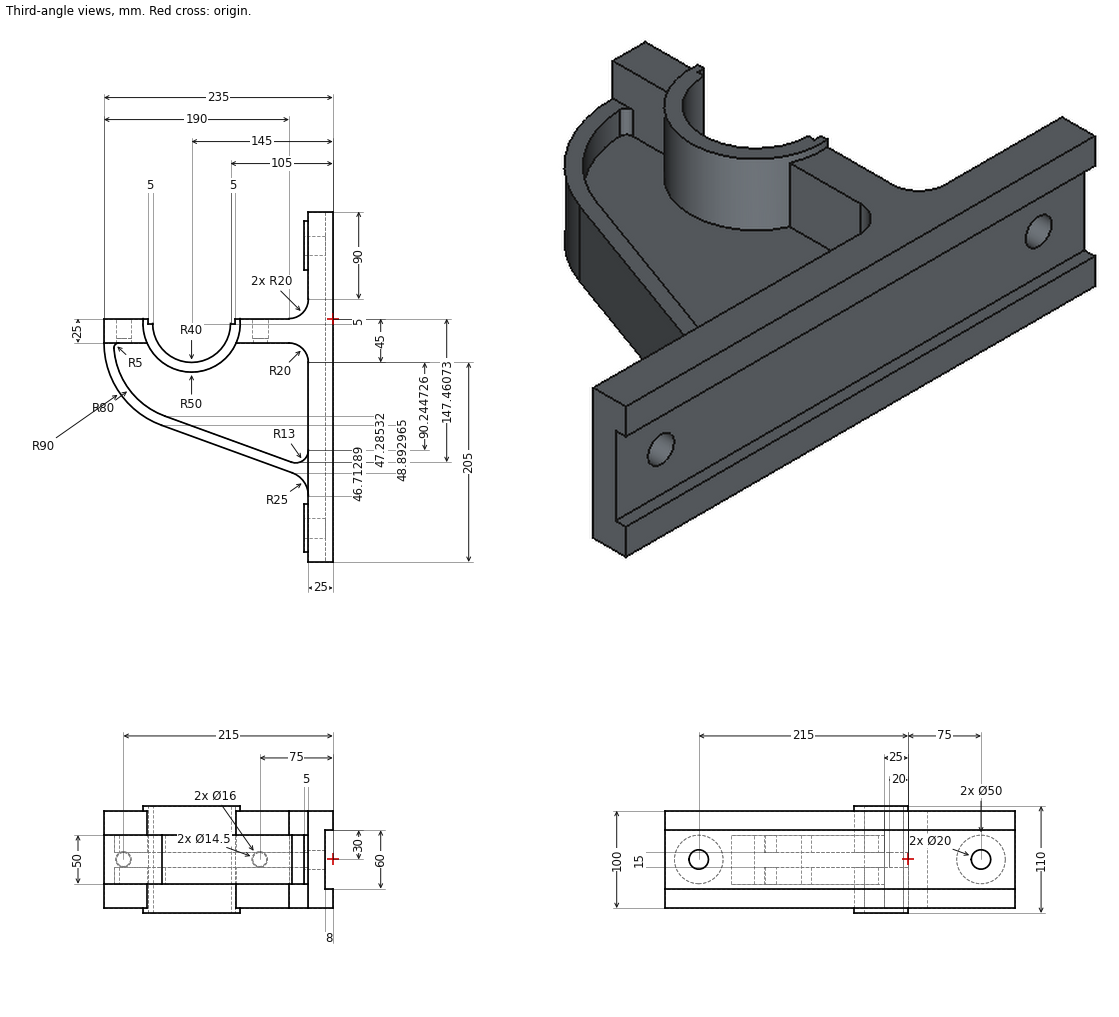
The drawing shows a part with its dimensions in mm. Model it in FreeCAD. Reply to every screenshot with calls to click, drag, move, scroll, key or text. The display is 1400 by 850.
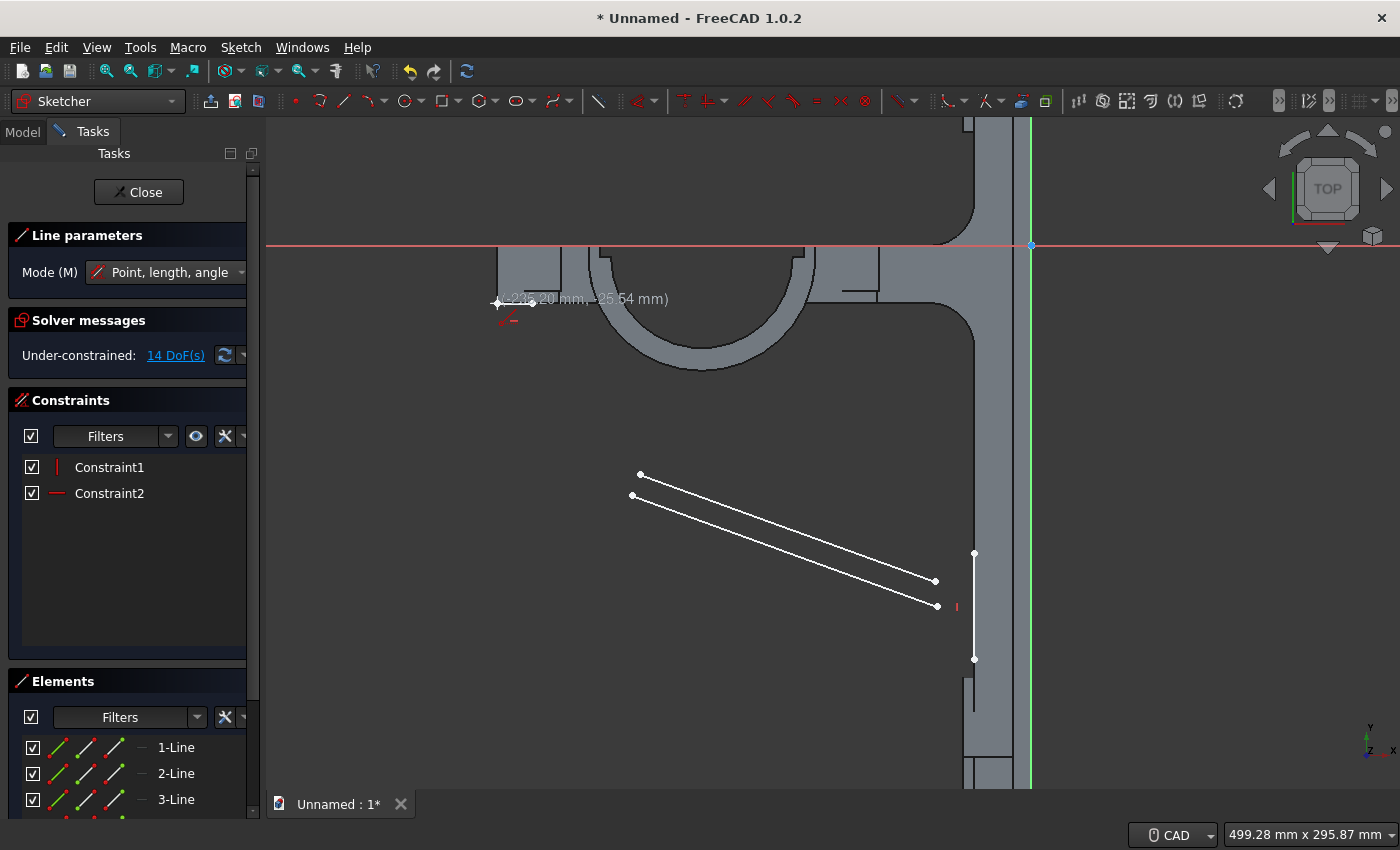
click(368, 102)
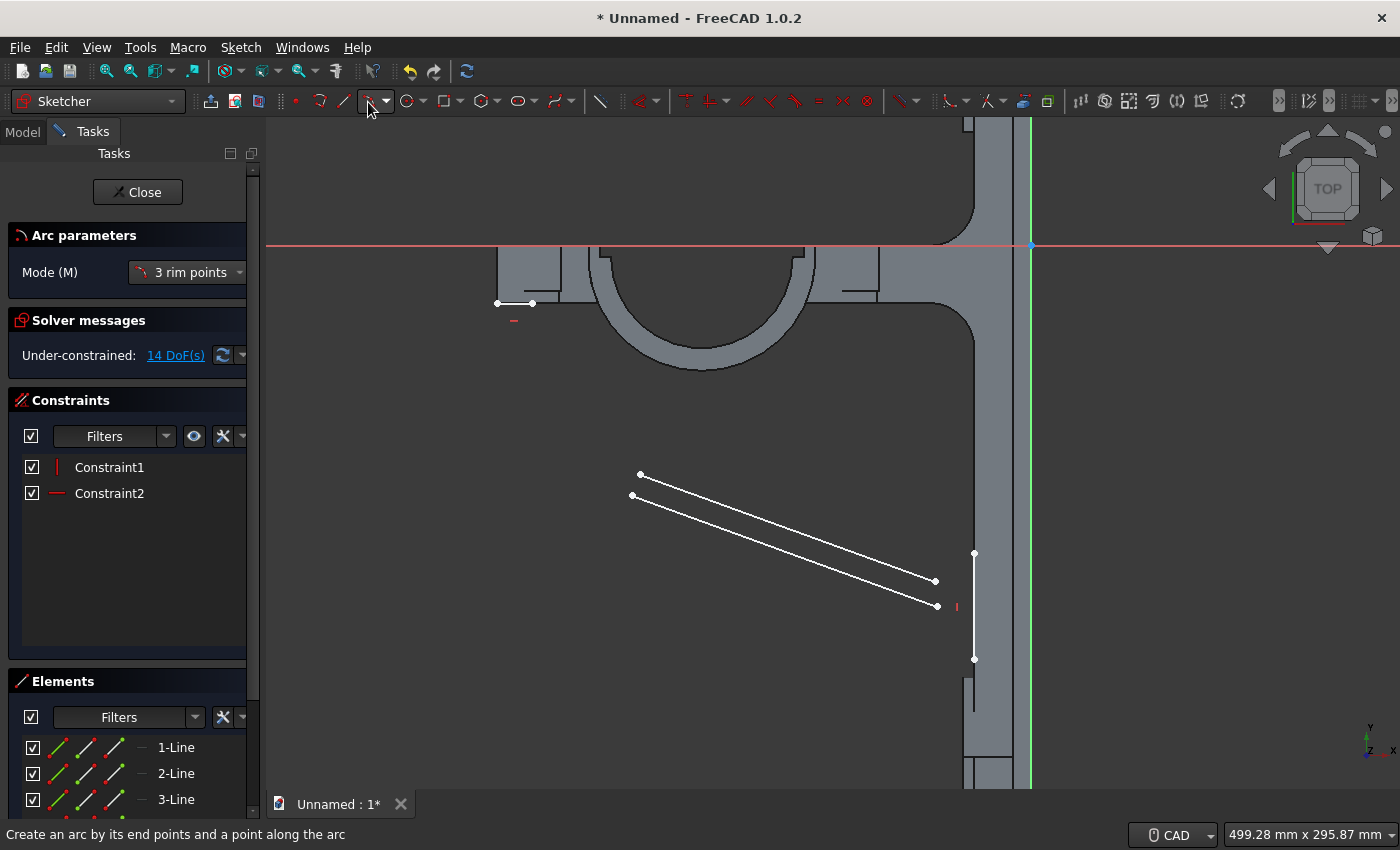
click(937, 607)
click(974, 660)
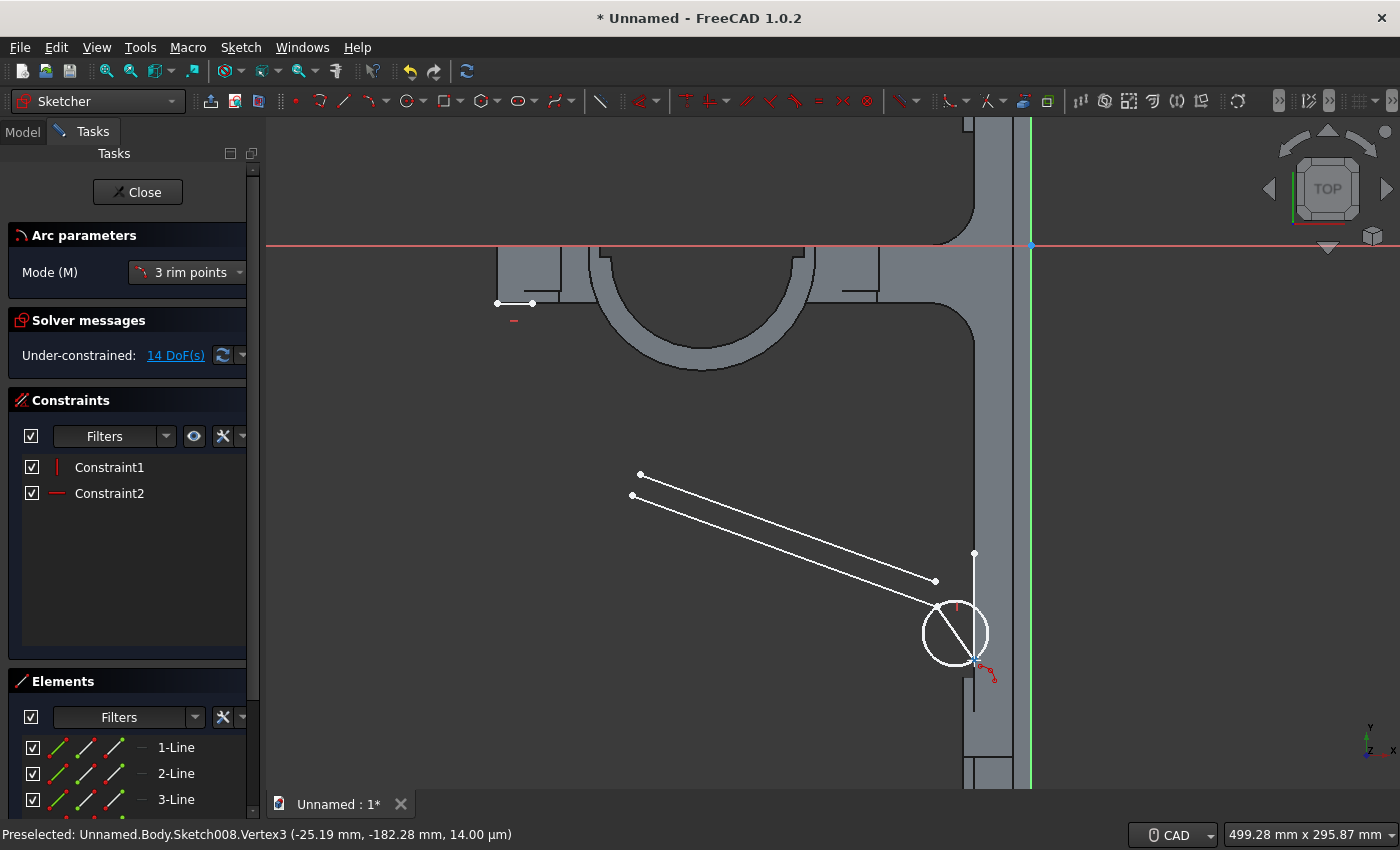
scroll(964, 627, up, 3)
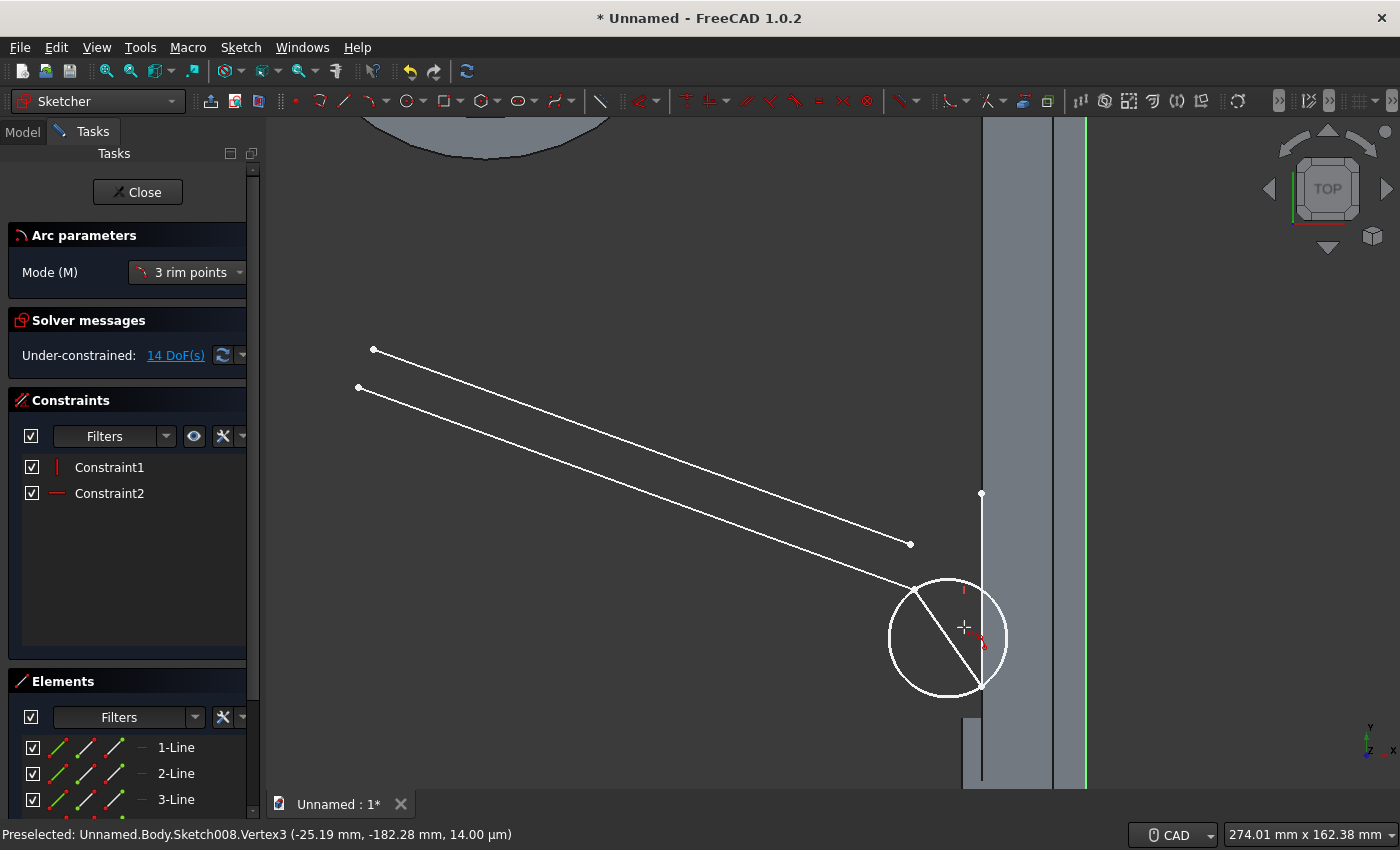
click(964, 626)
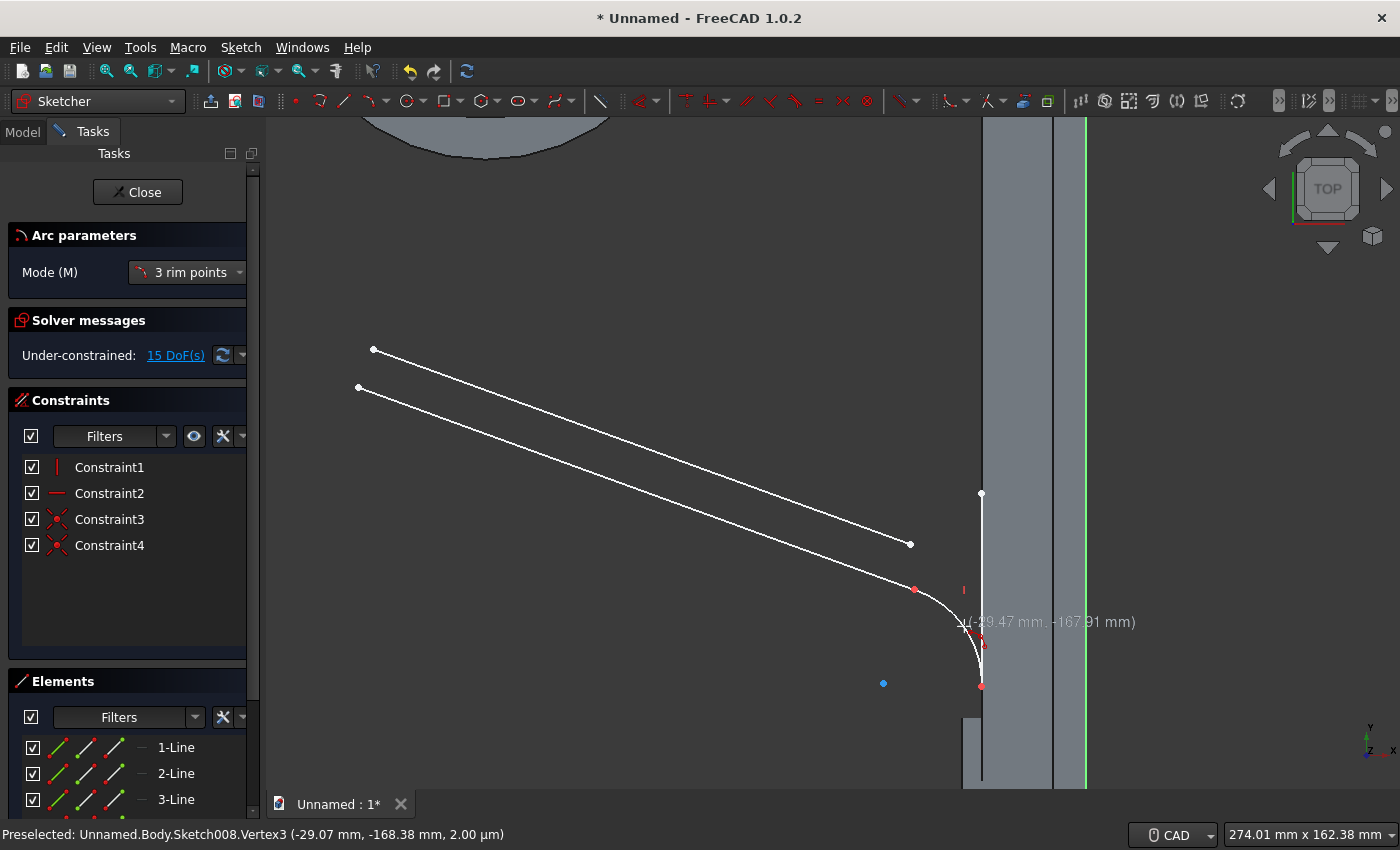
click(982, 493)
click(911, 544)
click(960, 536)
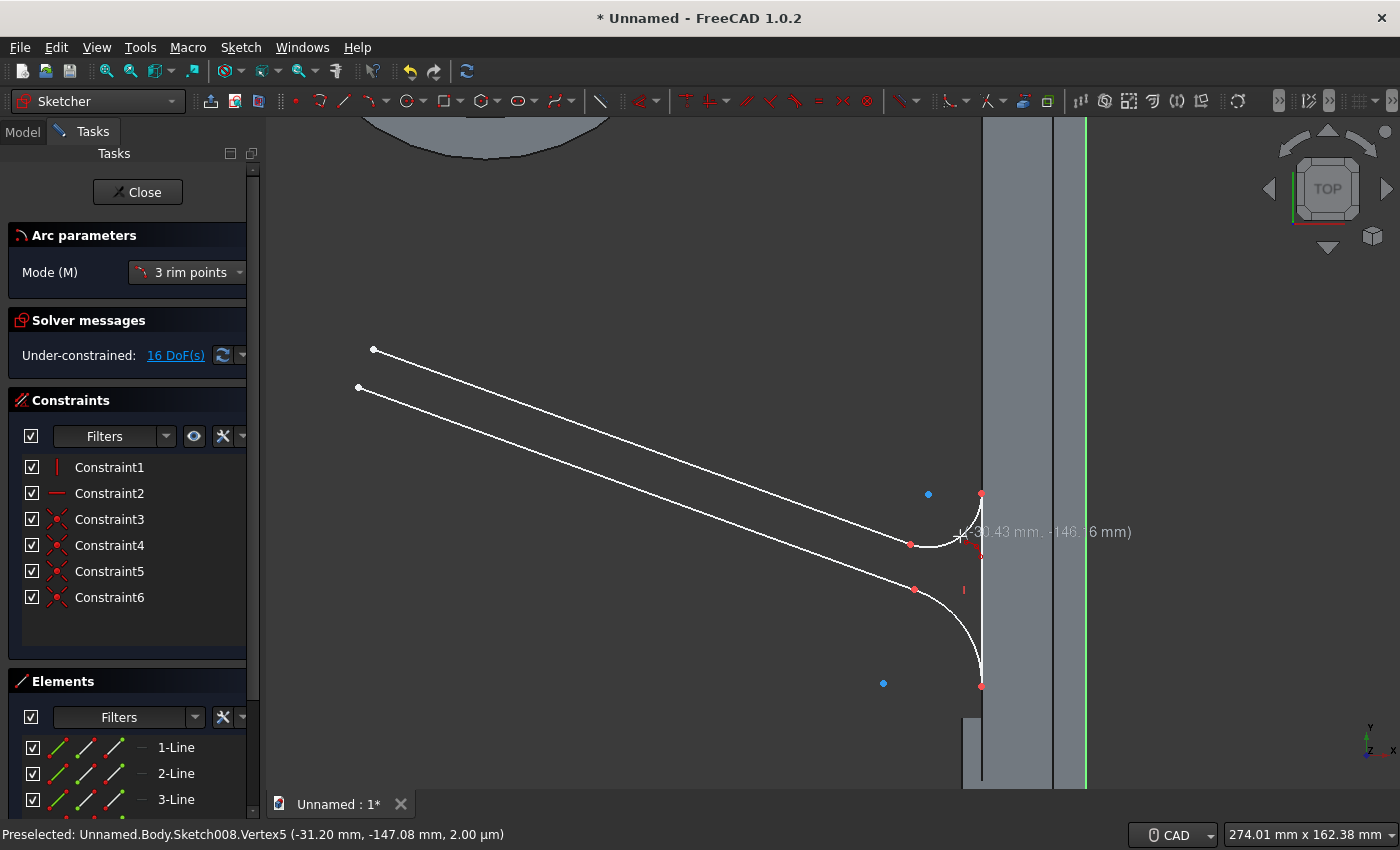
click(373, 349)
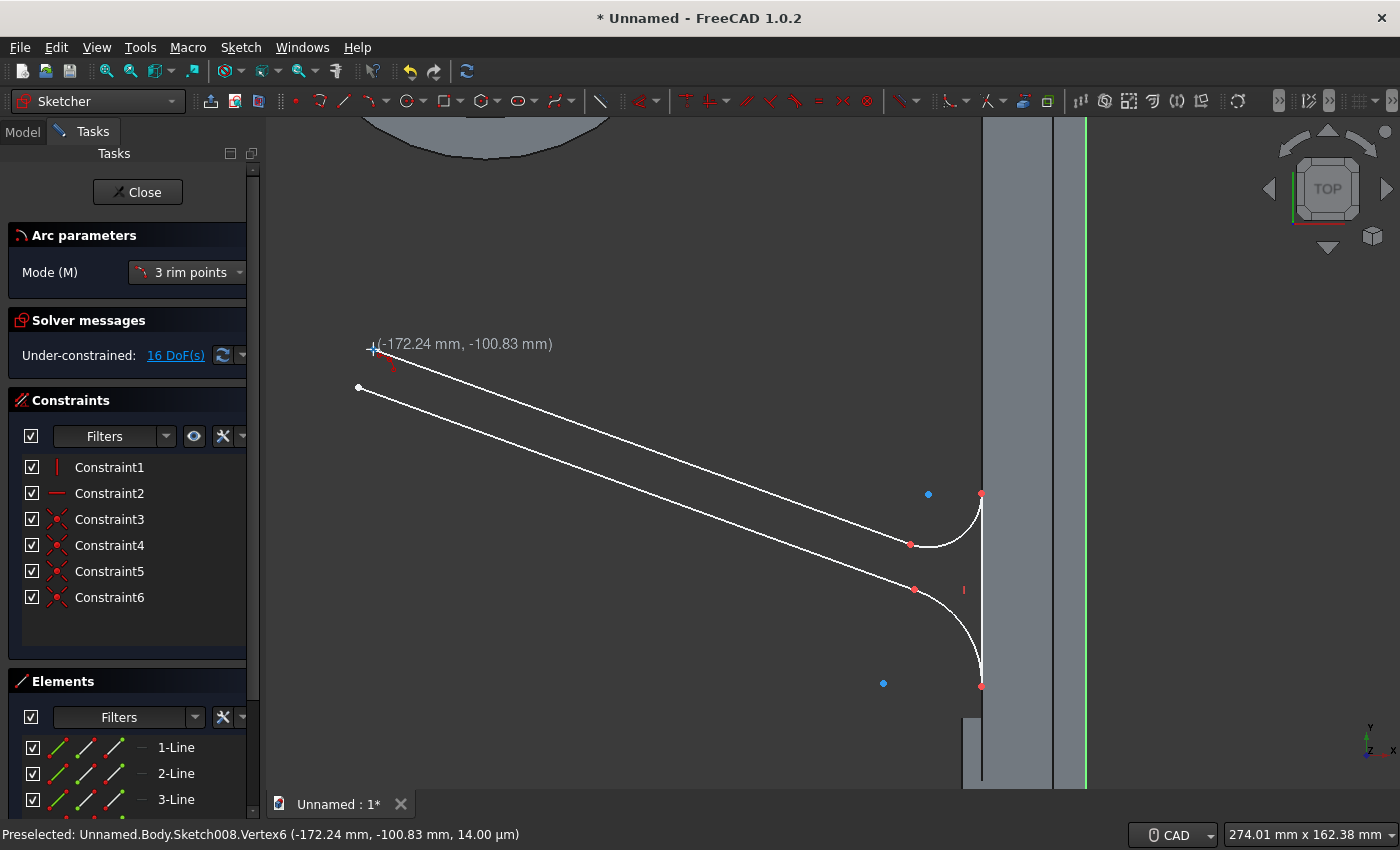
scroll(965, 629, down, 3)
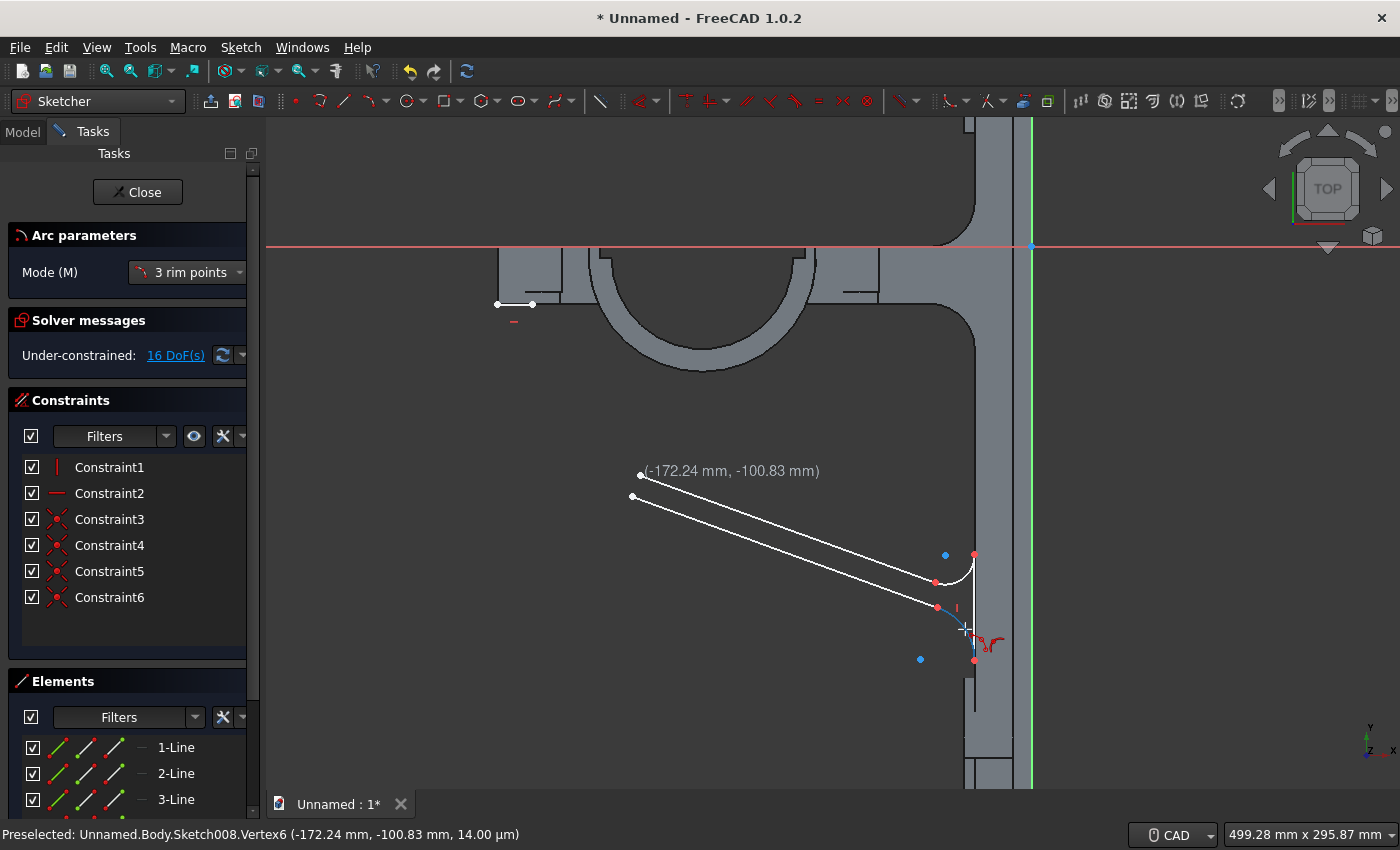
scroll(521, 316, up, 2)